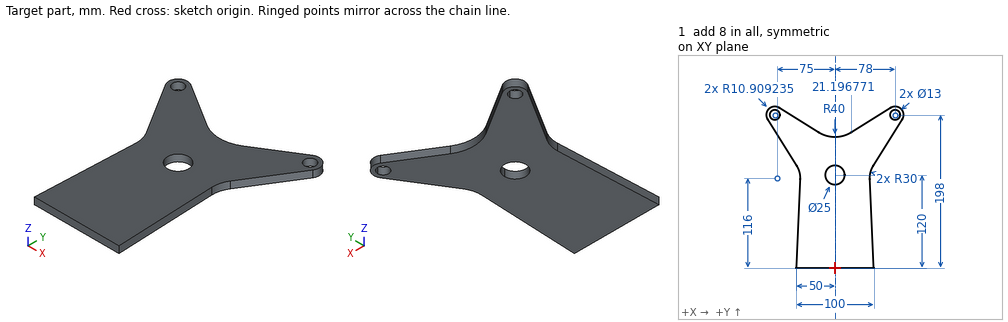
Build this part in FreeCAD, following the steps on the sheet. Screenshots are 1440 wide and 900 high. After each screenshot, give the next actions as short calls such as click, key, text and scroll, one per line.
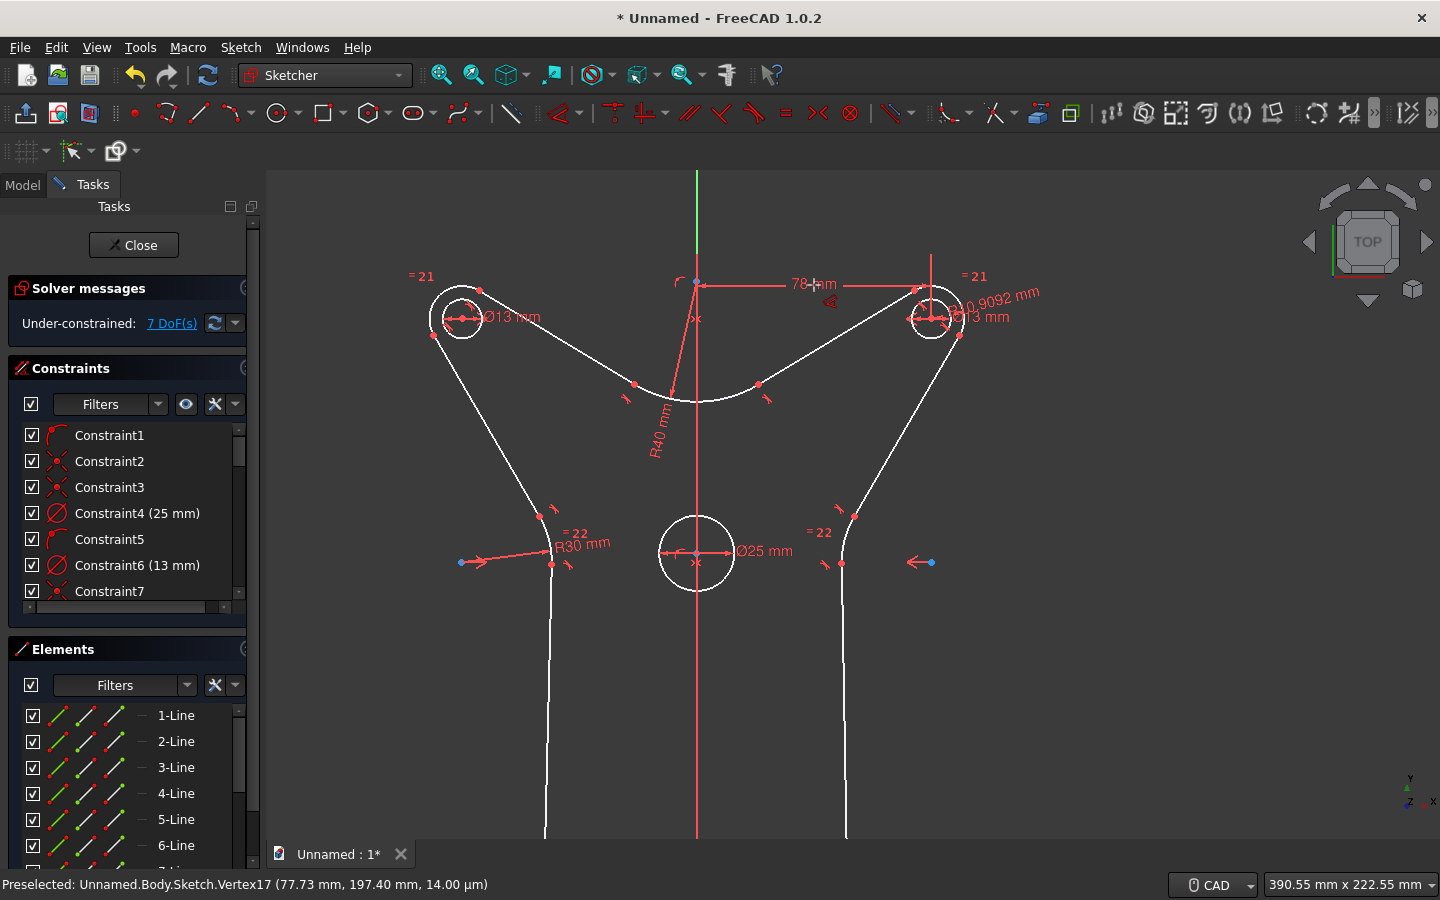
scroll(963, 309, down, 2)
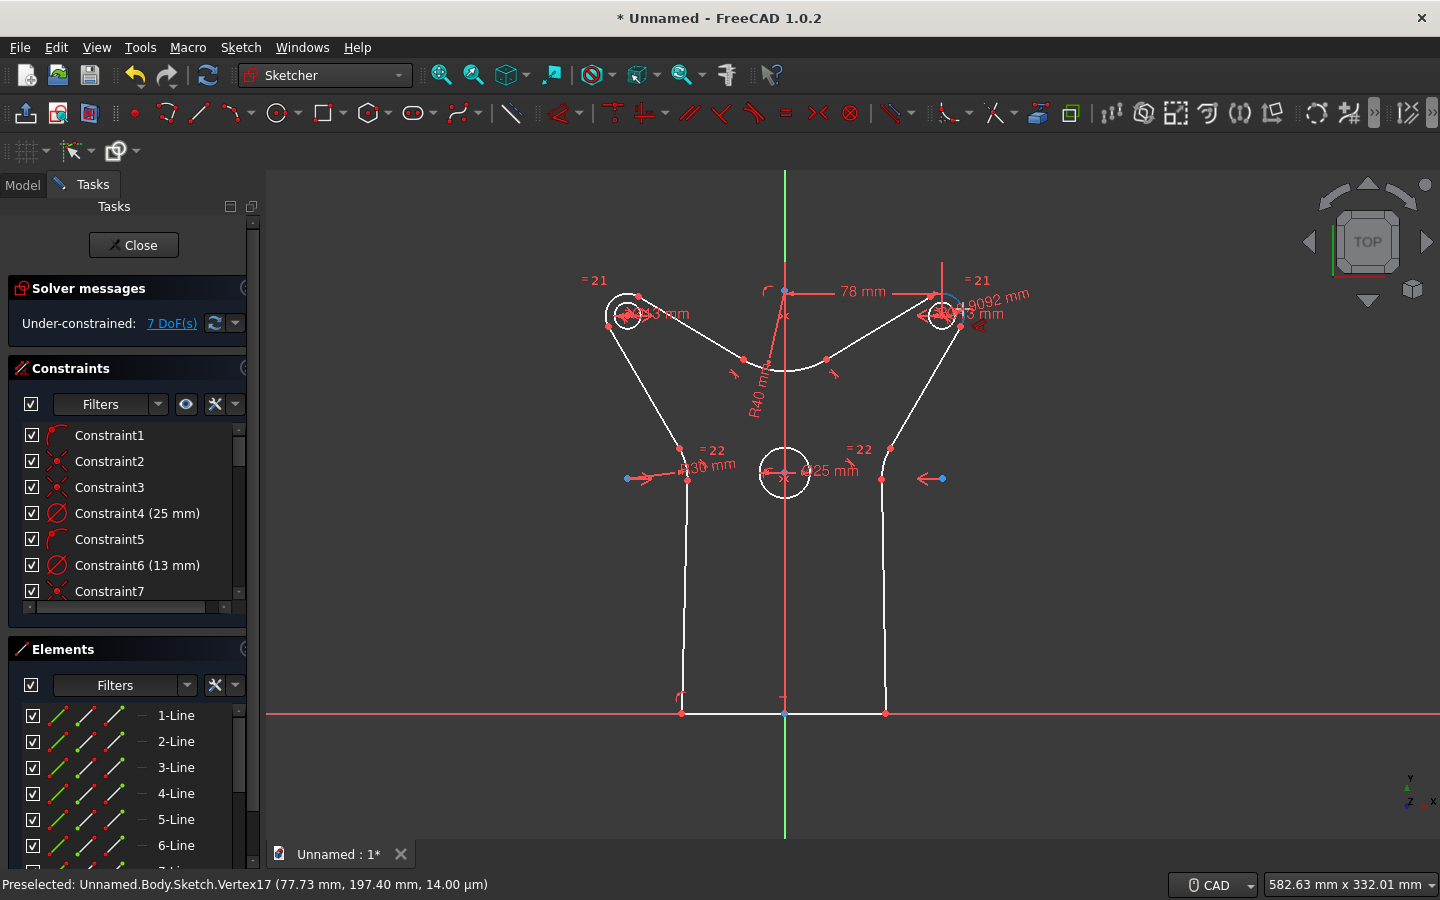
click(743, 714)
click(737, 748)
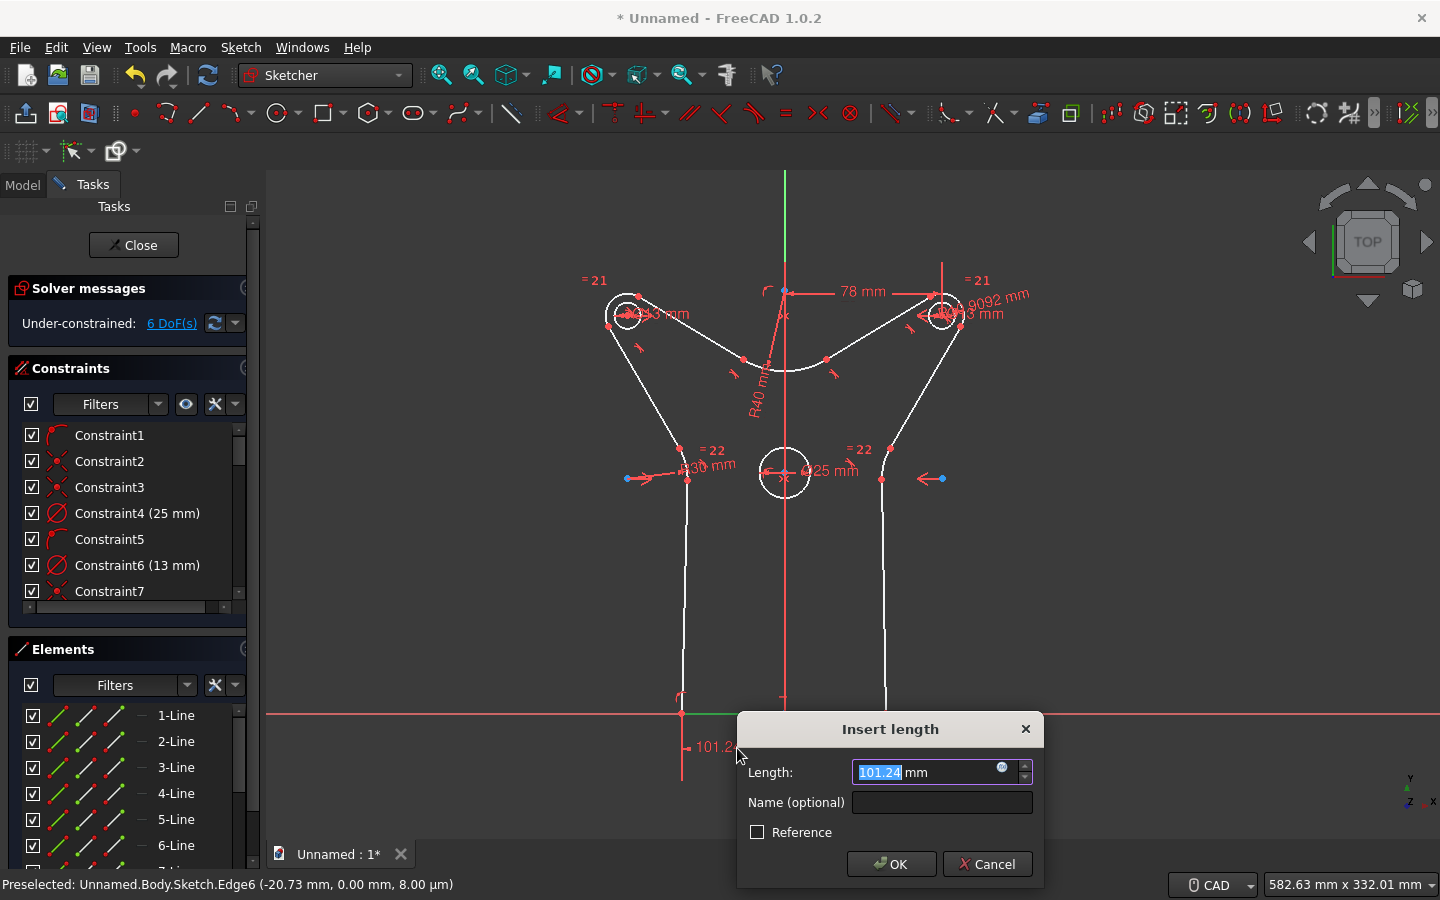
text(100)
key(Return)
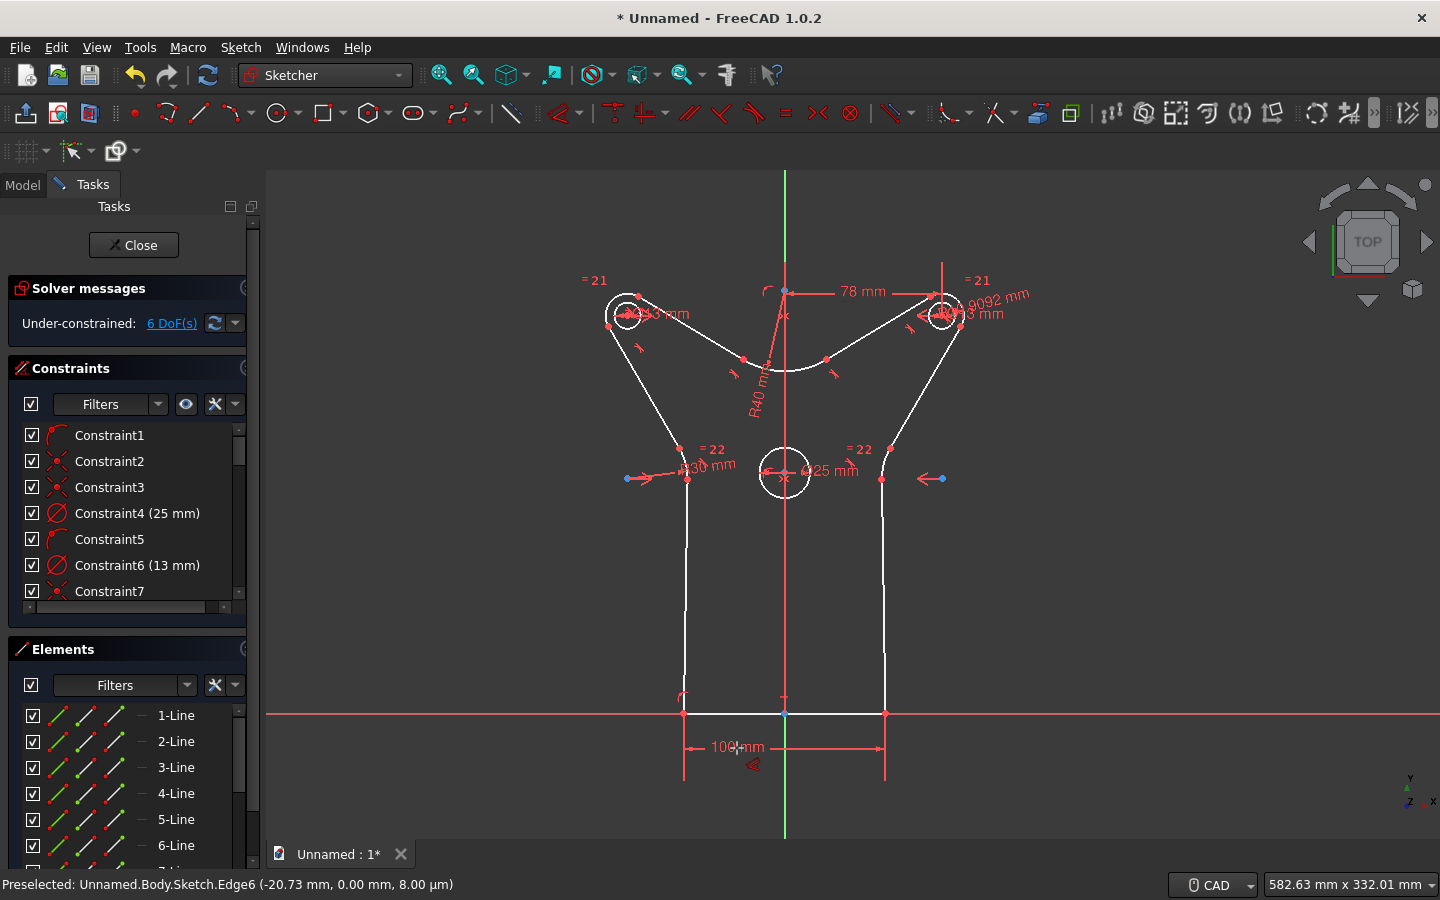
click(684, 714)
click(734, 680)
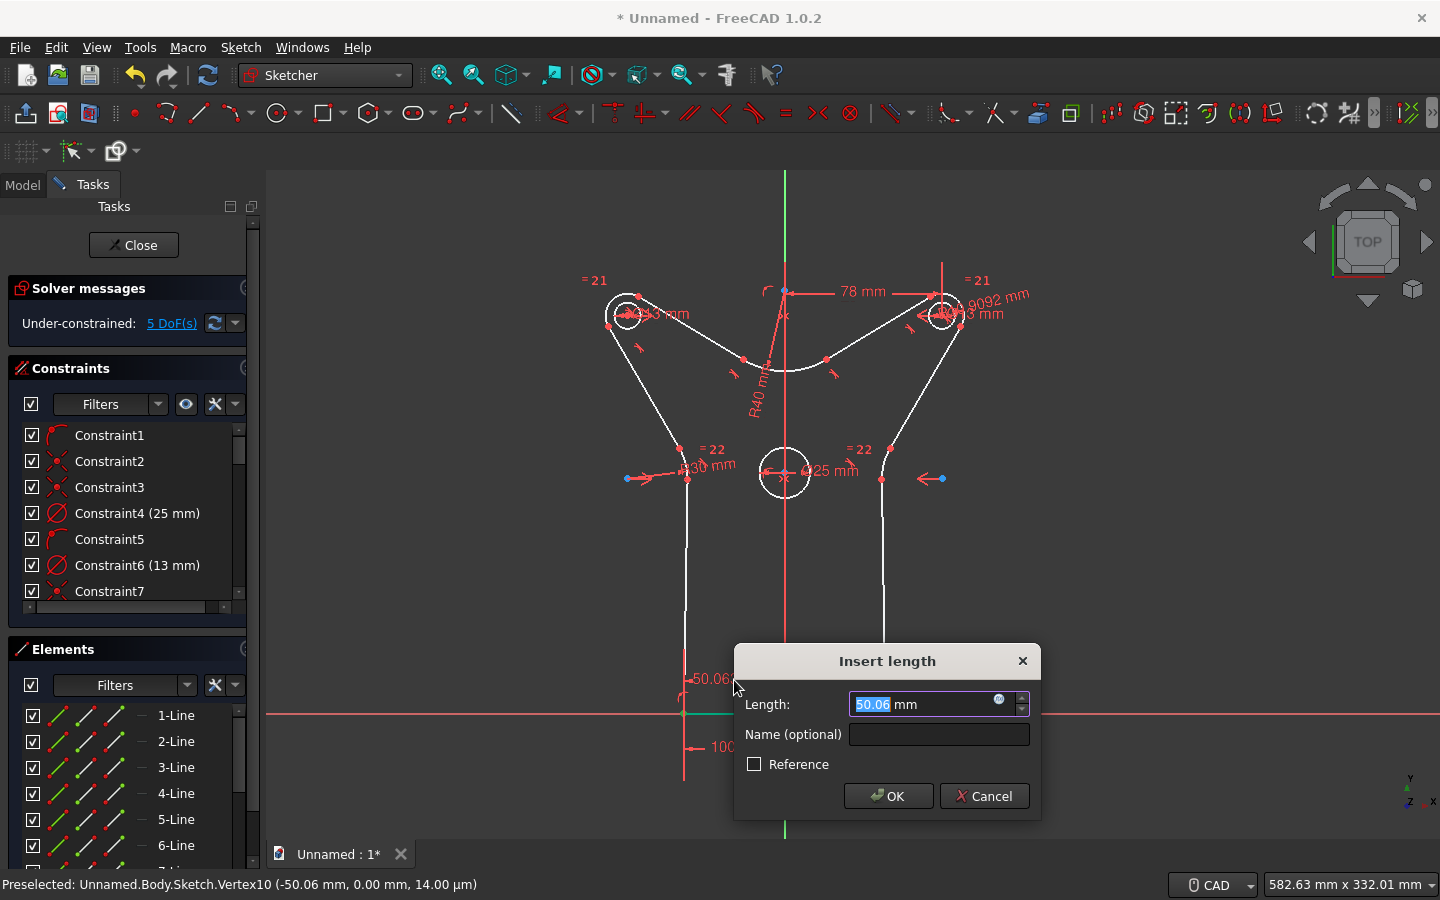
text(50)
key(Return)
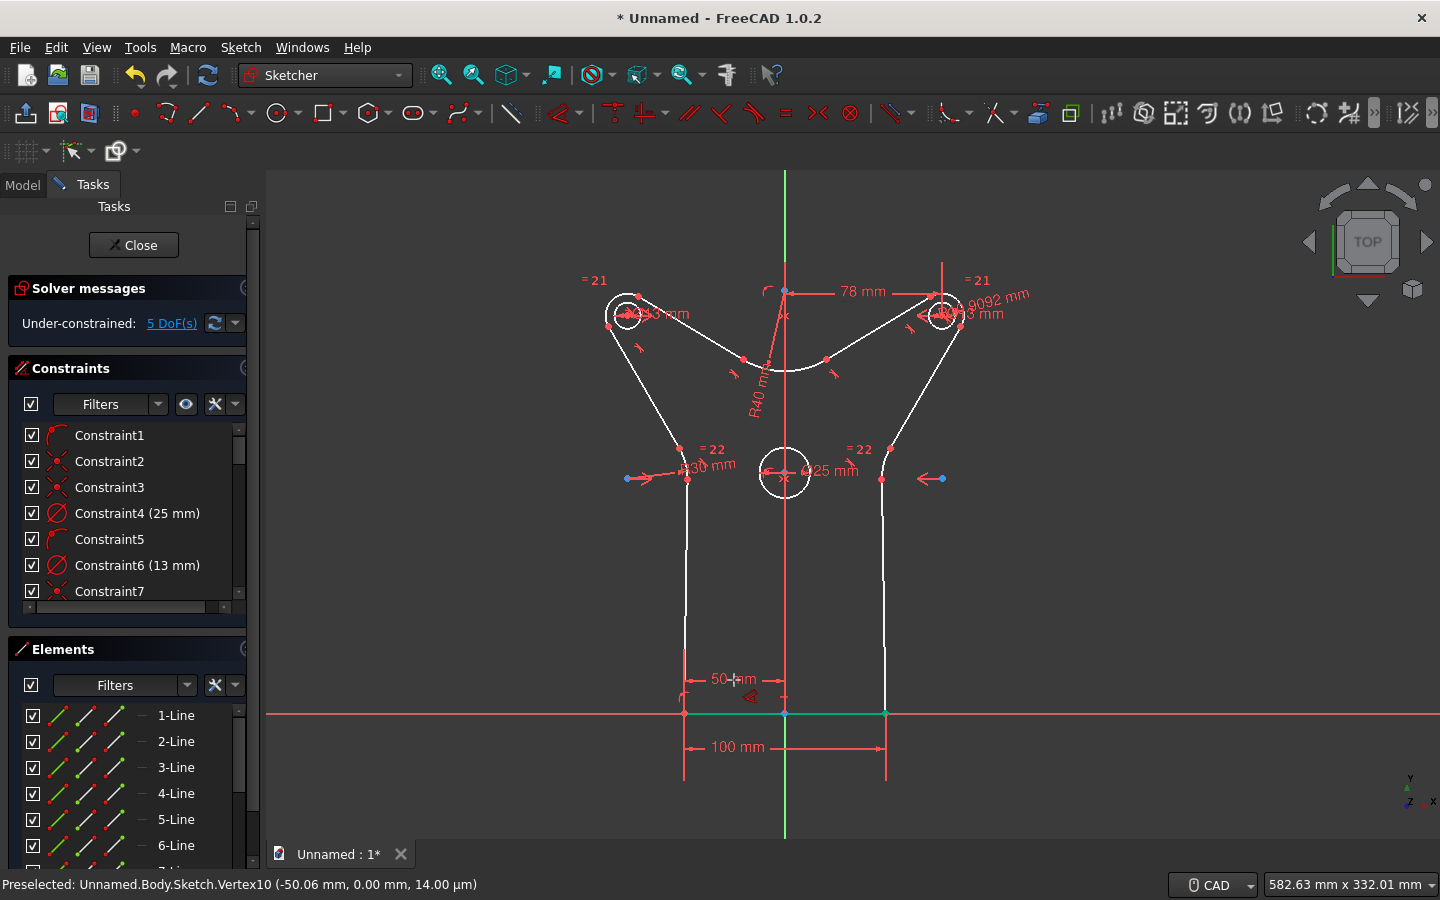
click(627, 479)
click(651, 748)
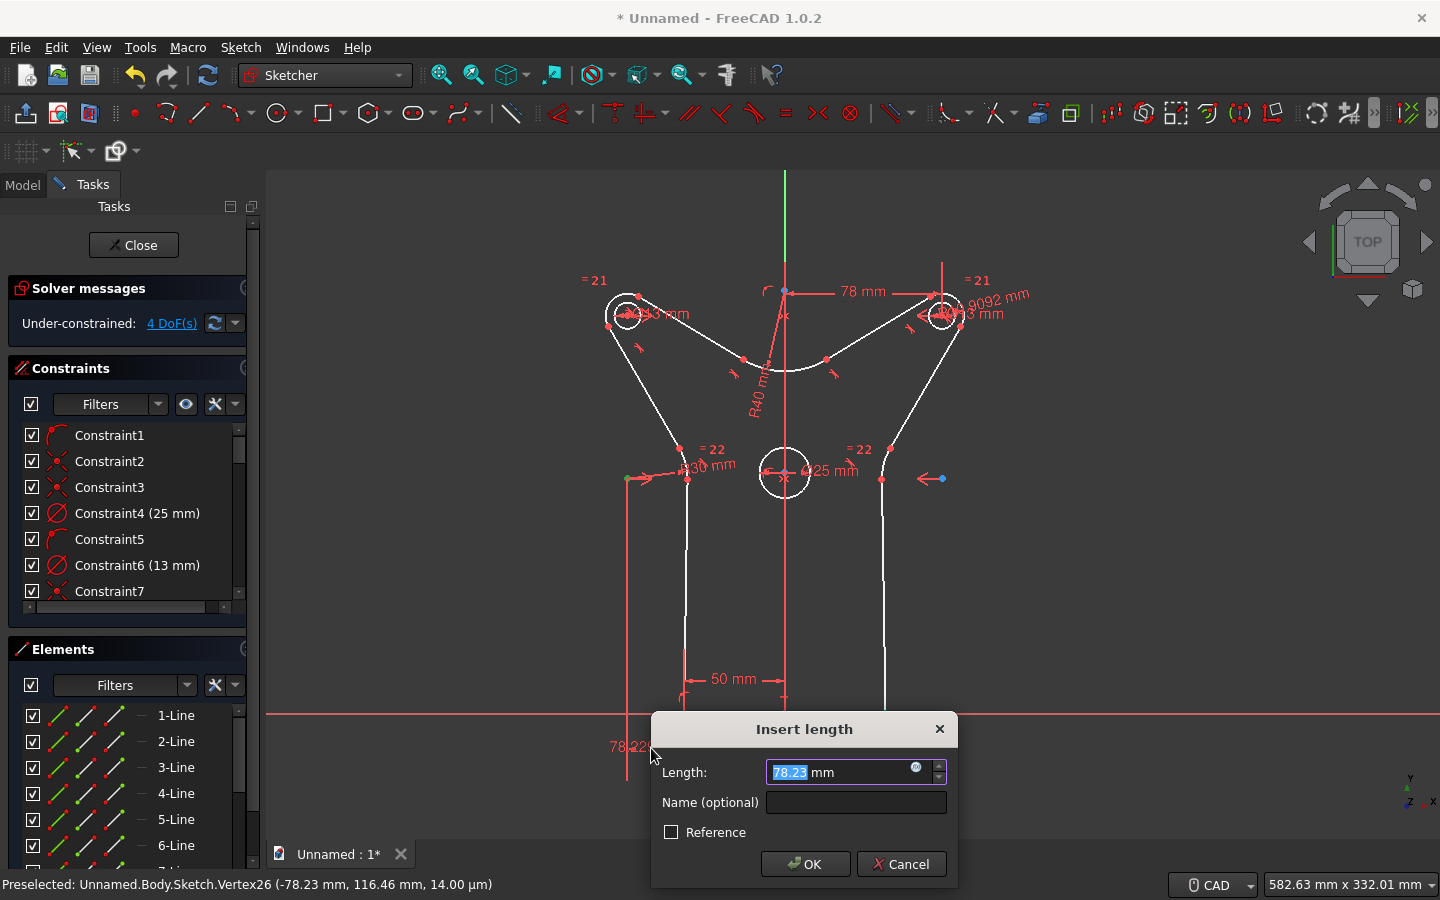
text(75)
key(Return)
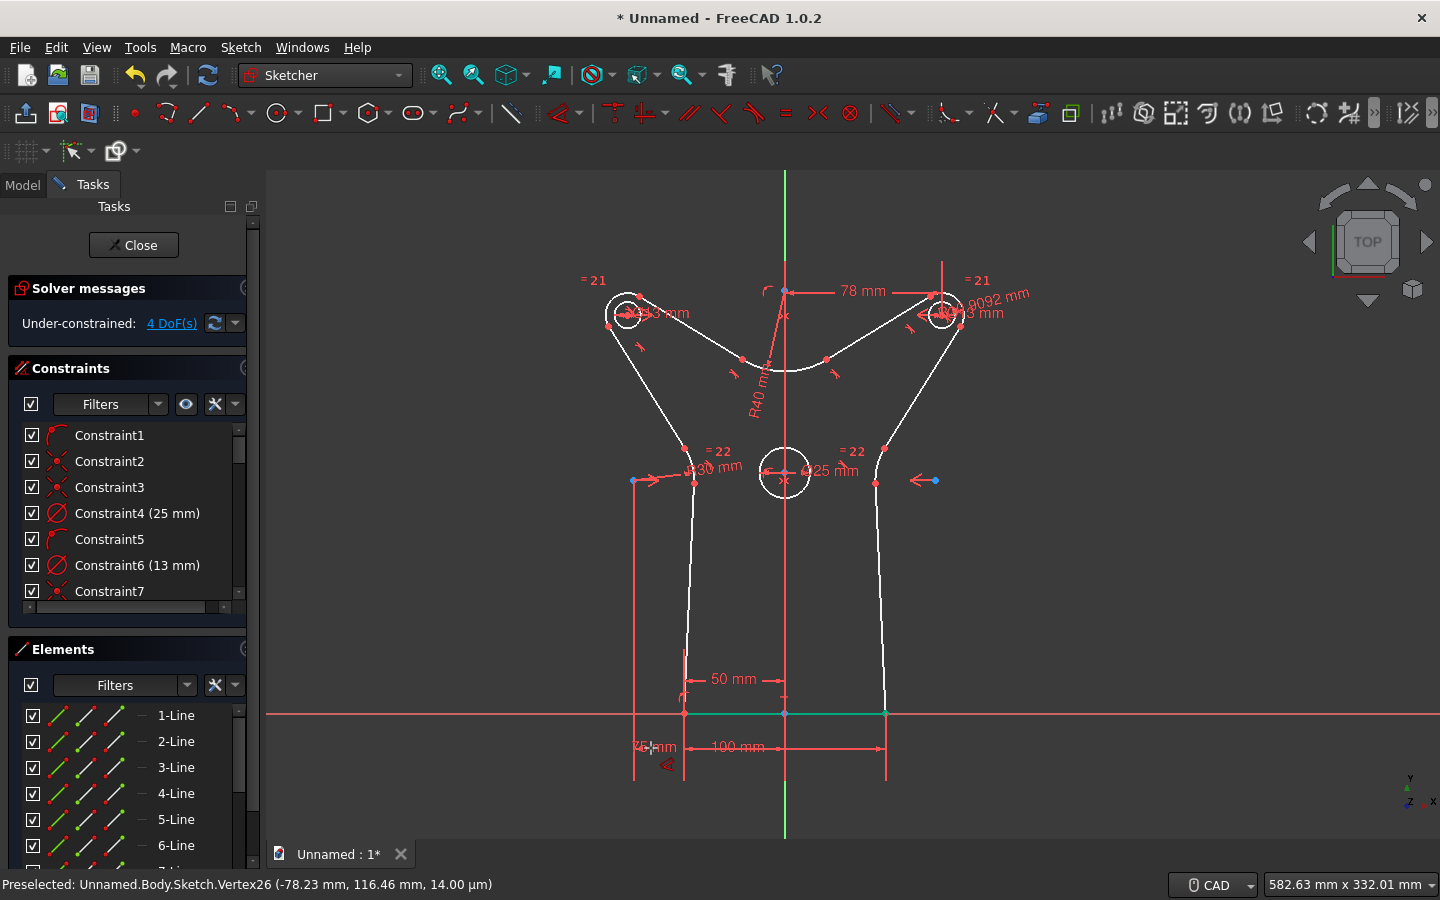
click(785, 473)
click(819, 593)